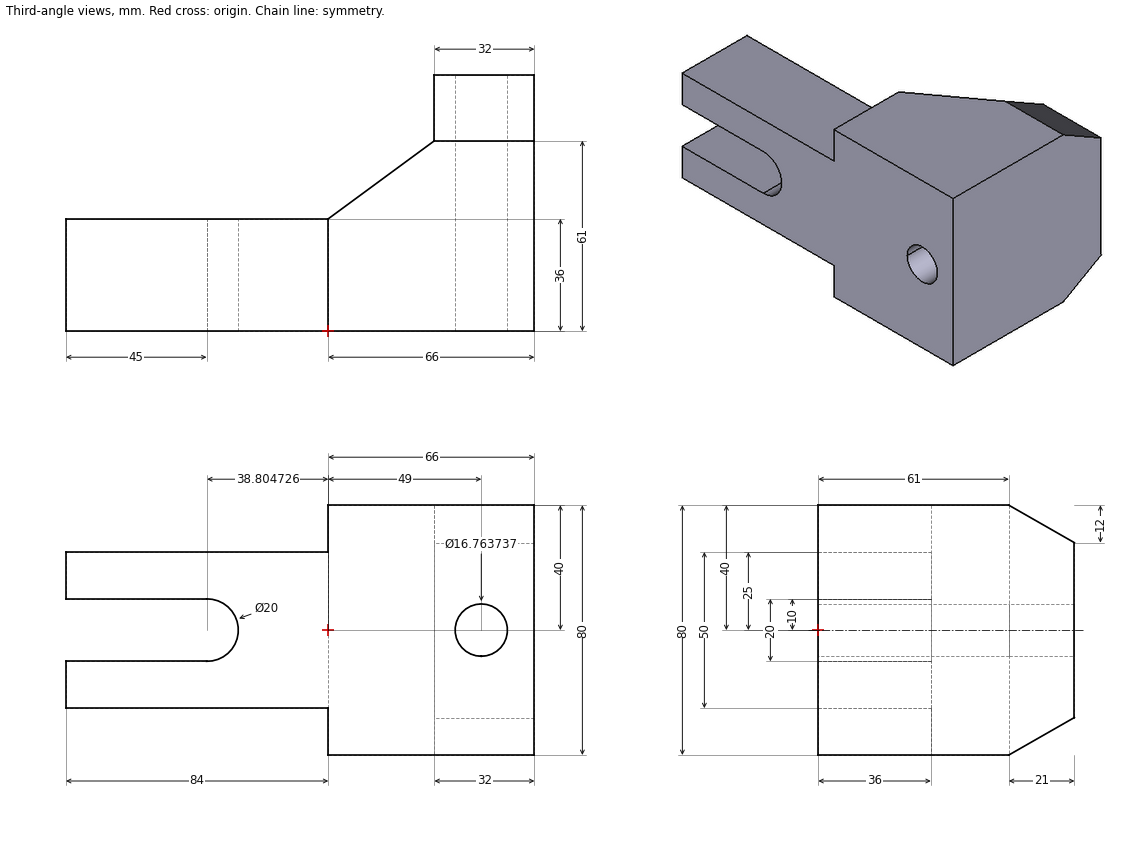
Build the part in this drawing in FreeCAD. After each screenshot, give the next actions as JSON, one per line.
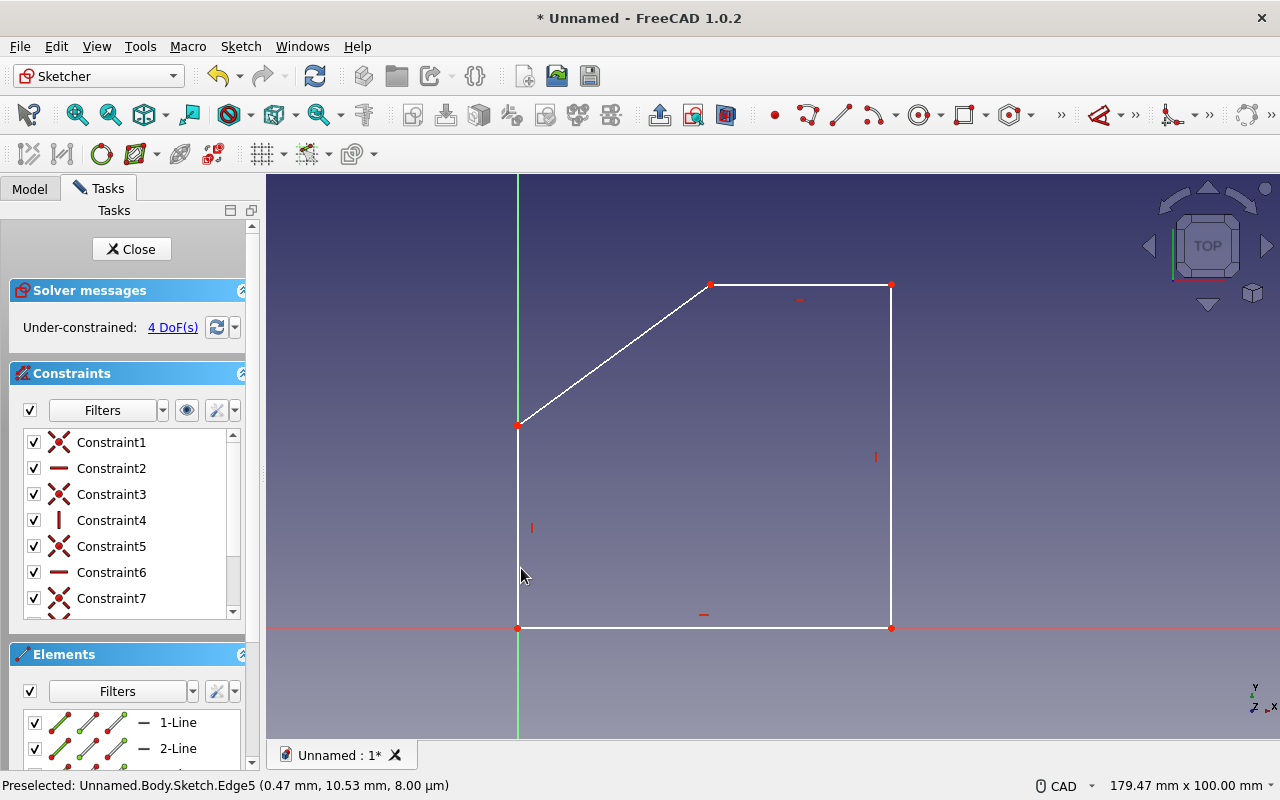
{"action": "key", "text": "d"}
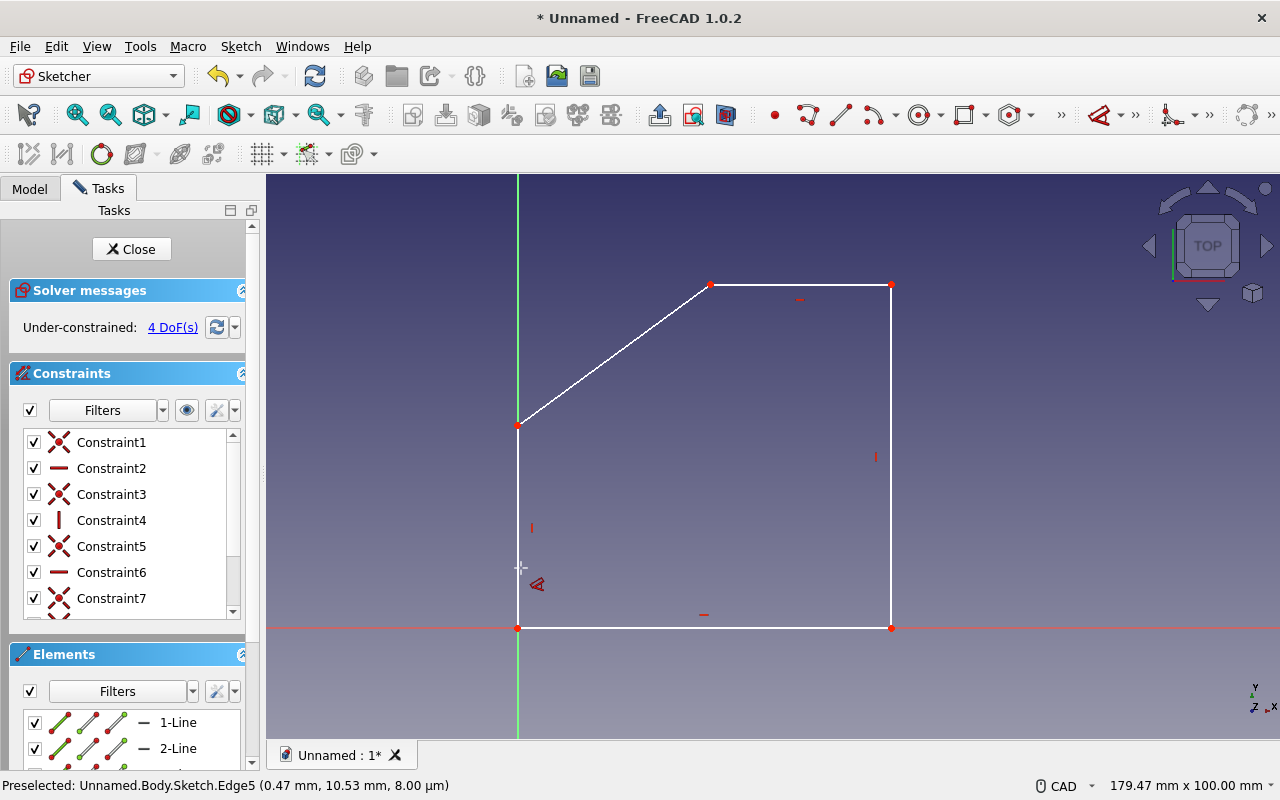
{"action": "left_click", "coordinate": [630, 628]}
{"action": "left_click", "coordinate": [704, 662]}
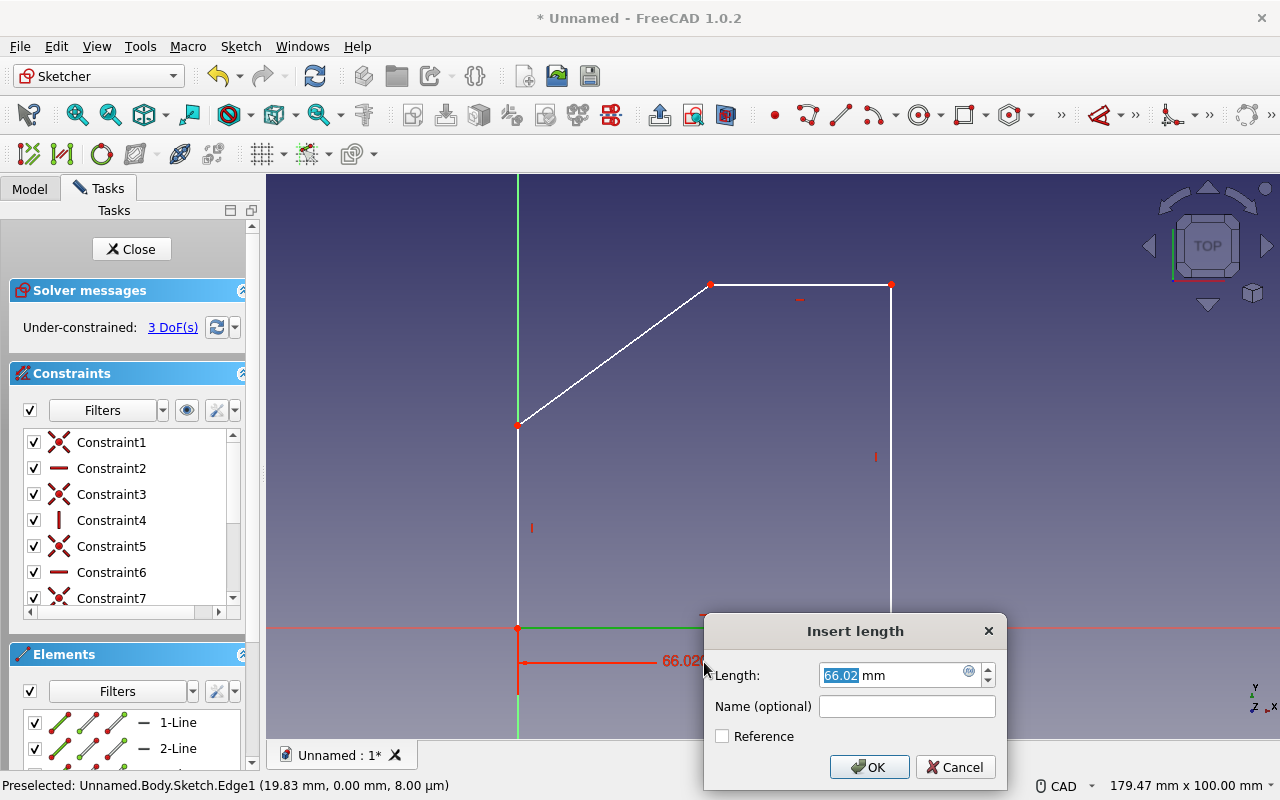
{"action": "type", "text": "66"}
{"action": "key", "text": "Return"}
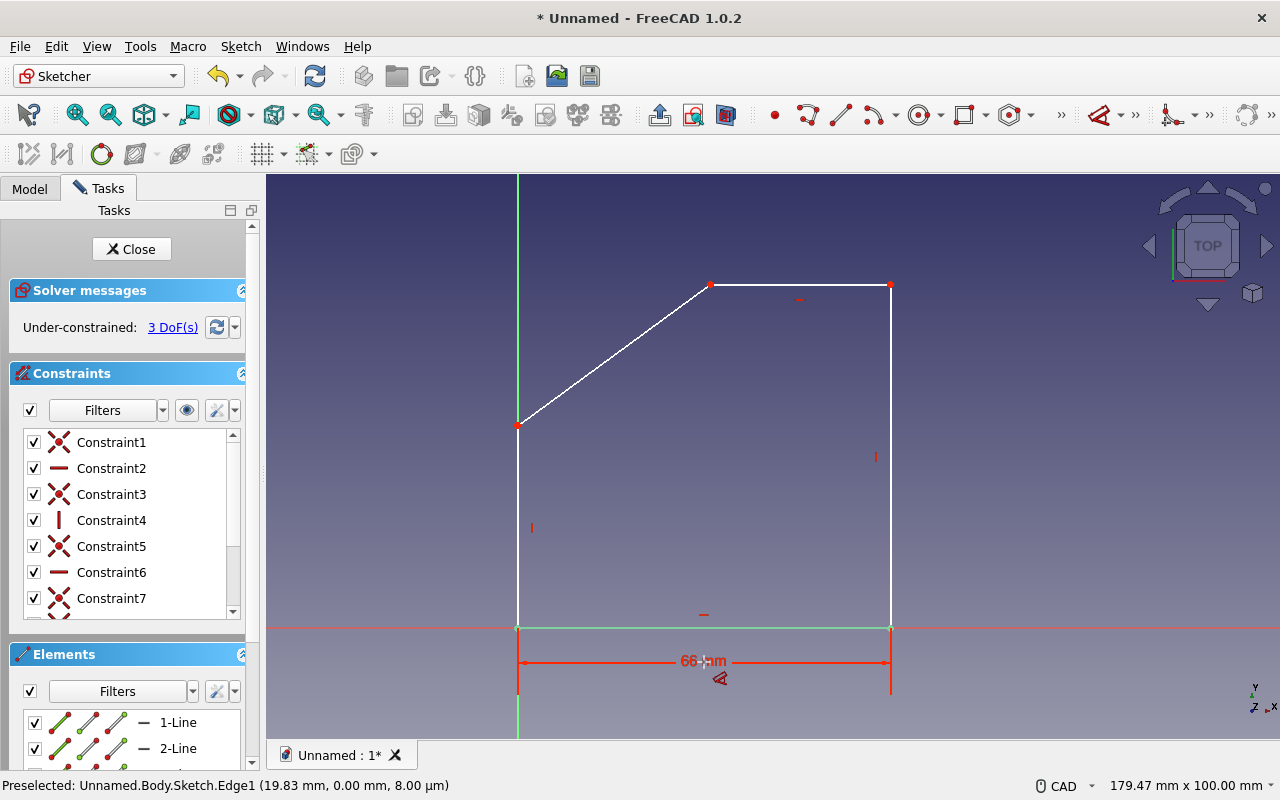
{"action": "left_click", "coordinate": [891, 525]}
{"action": "left_click", "coordinate": [925, 457]}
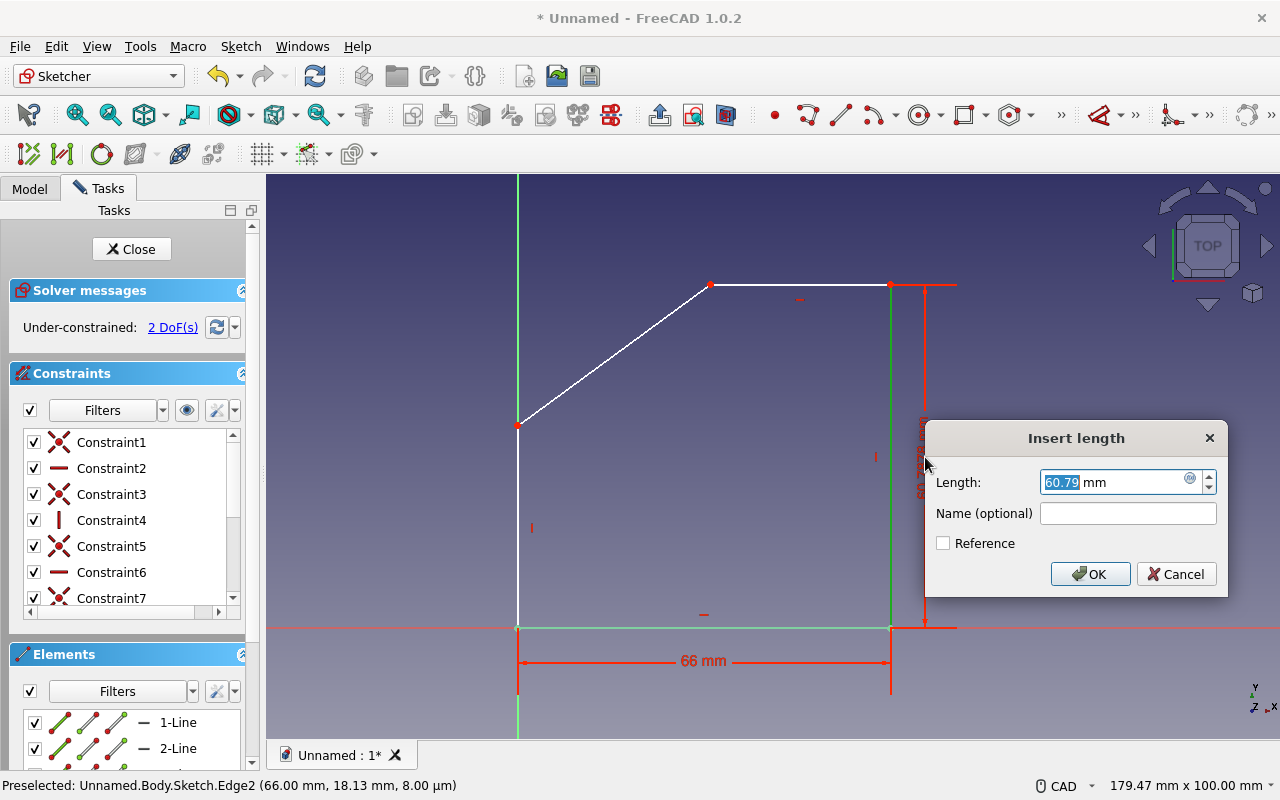
{"action": "type", "text": "61"}
{"action": "key", "text": "Return"}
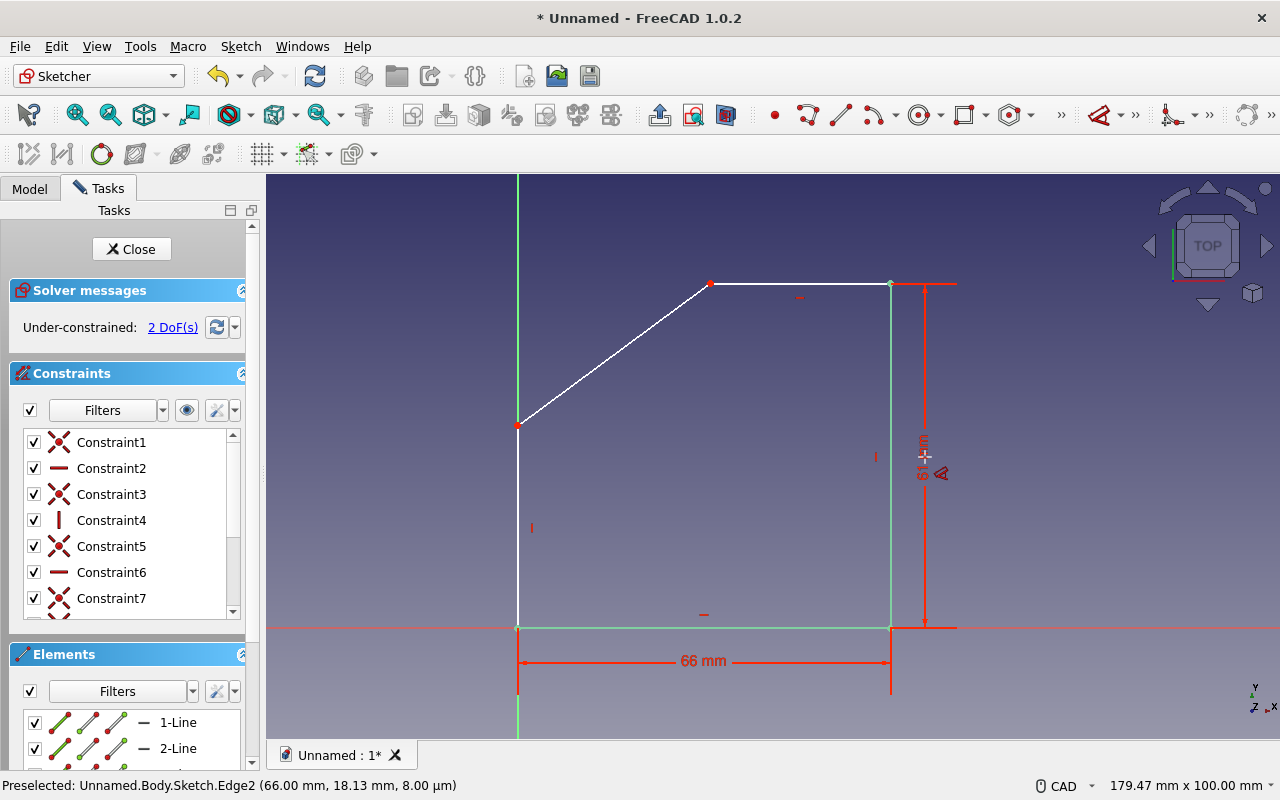
{"action": "left_click", "coordinate": [837, 284]}
{"action": "left_click", "coordinate": [800, 250]}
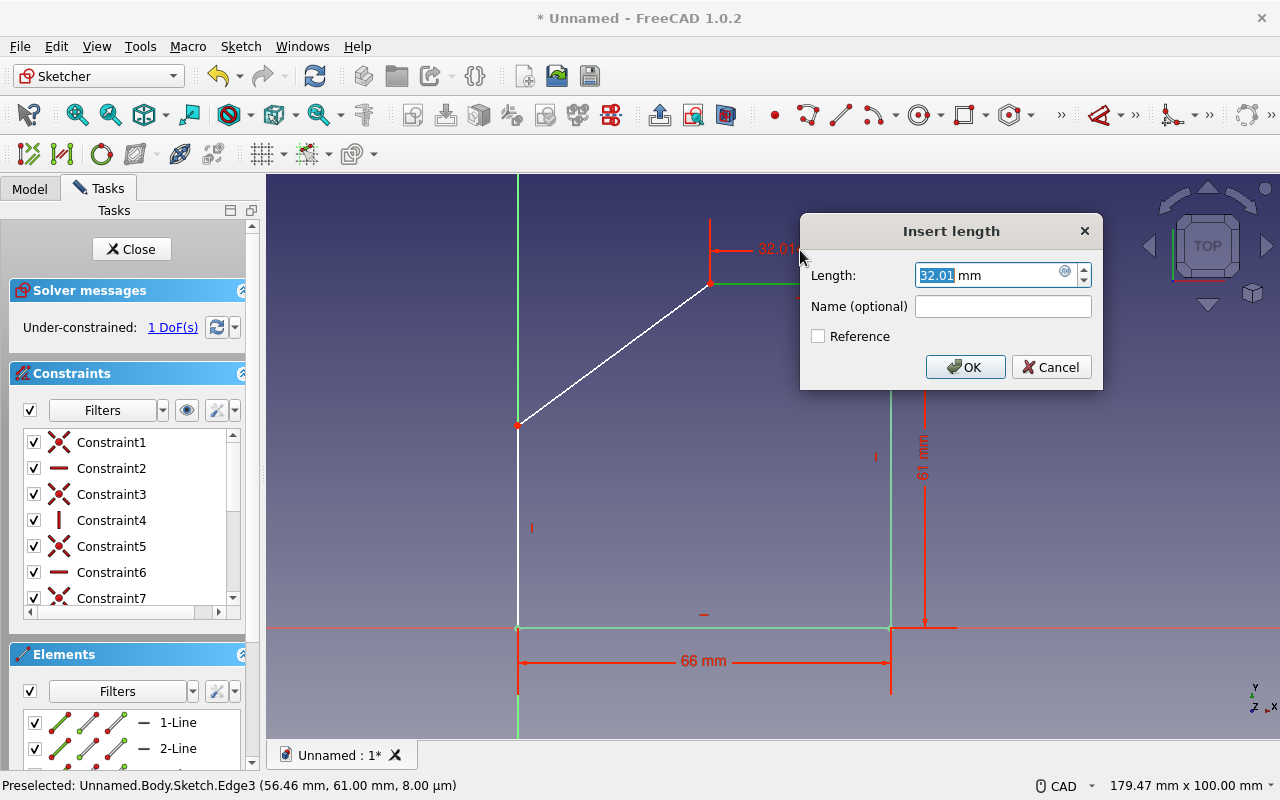
{"action": "type", "text": "32"}
{"action": "key", "text": "Return"}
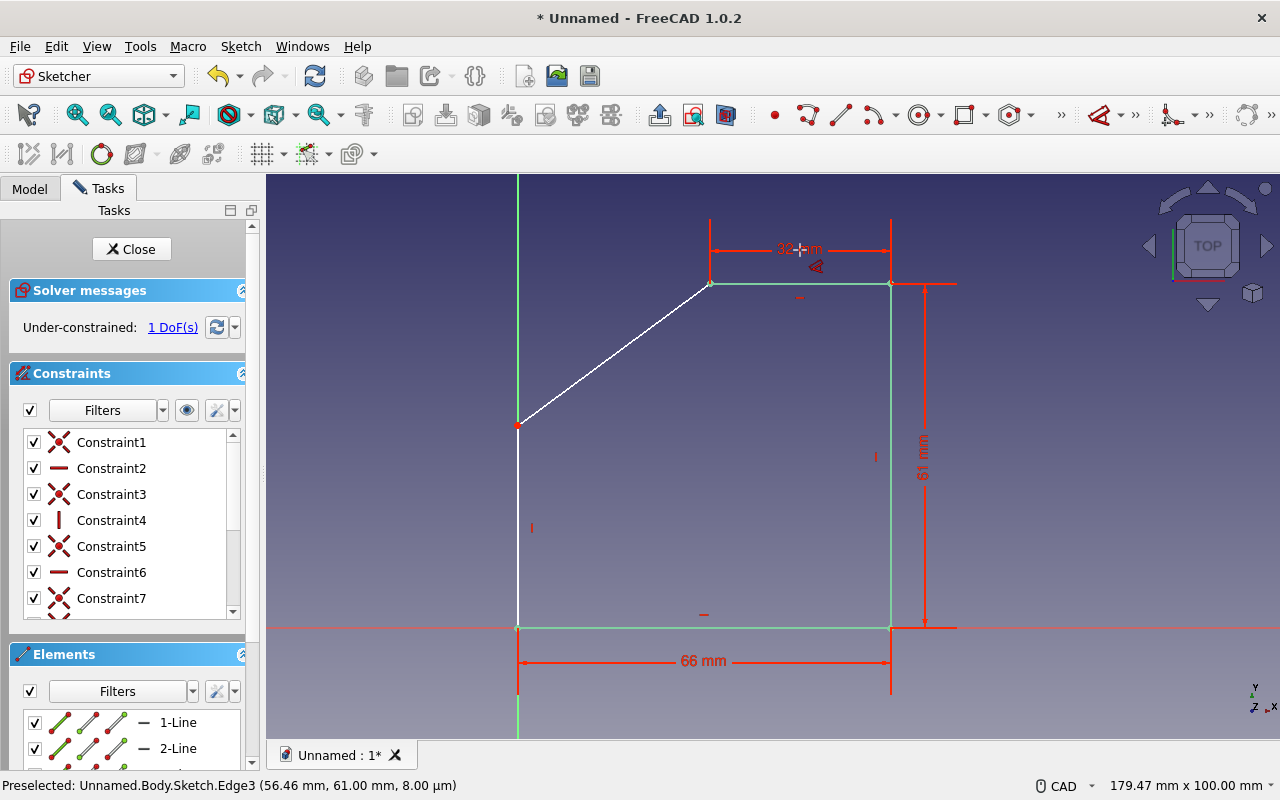
{"action": "left_click", "coordinate": [518, 487]}
{"action": "left_click", "coordinate": [484, 527]}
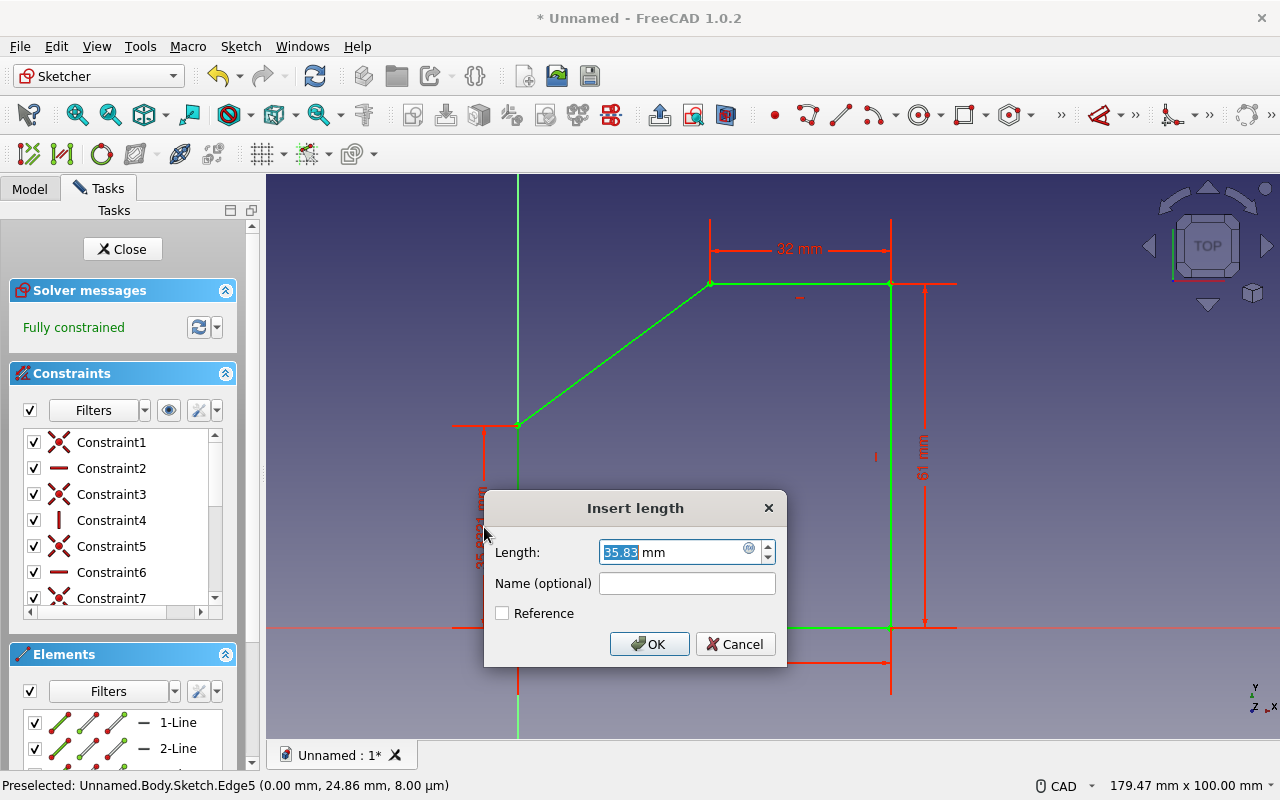
{"action": "type", "text": "36"}
{"action": "key", "text": "Return"}
{"action": "key", "text": "Escape"}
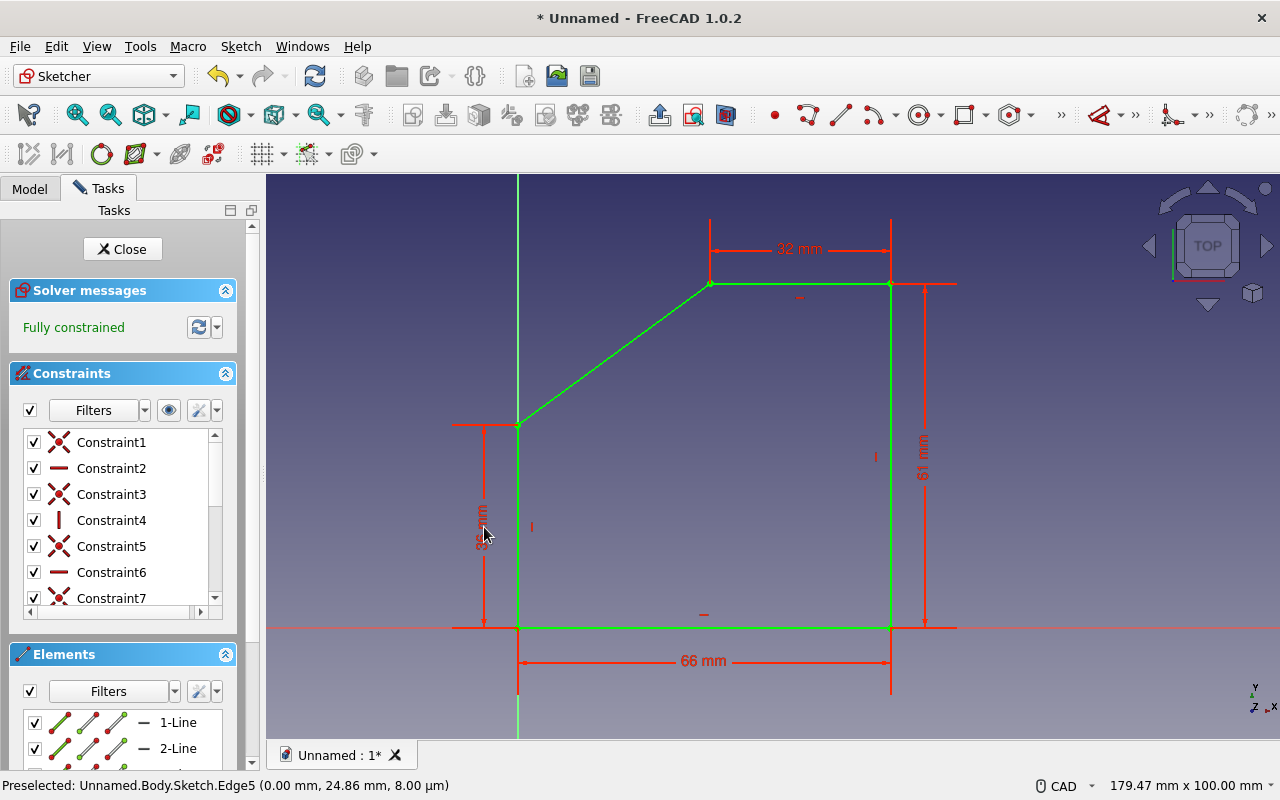
{"action": "left_click", "coordinate": [123, 249]}